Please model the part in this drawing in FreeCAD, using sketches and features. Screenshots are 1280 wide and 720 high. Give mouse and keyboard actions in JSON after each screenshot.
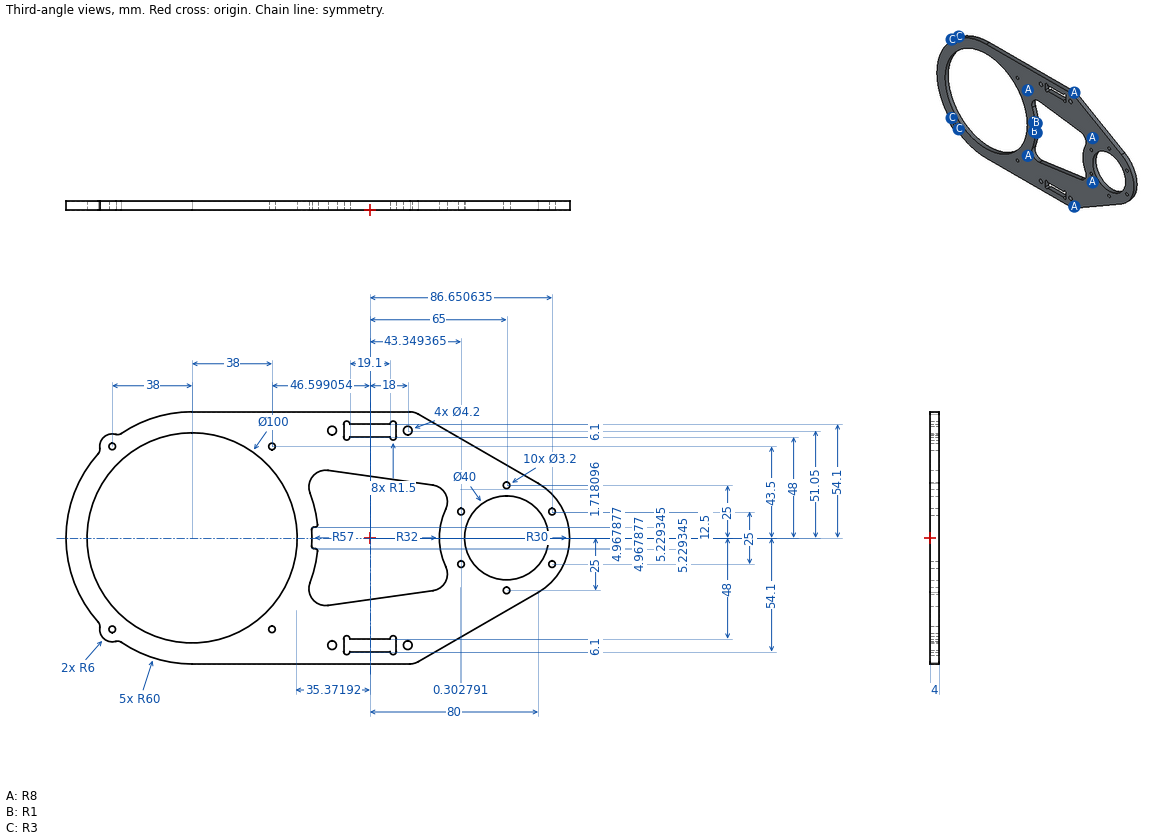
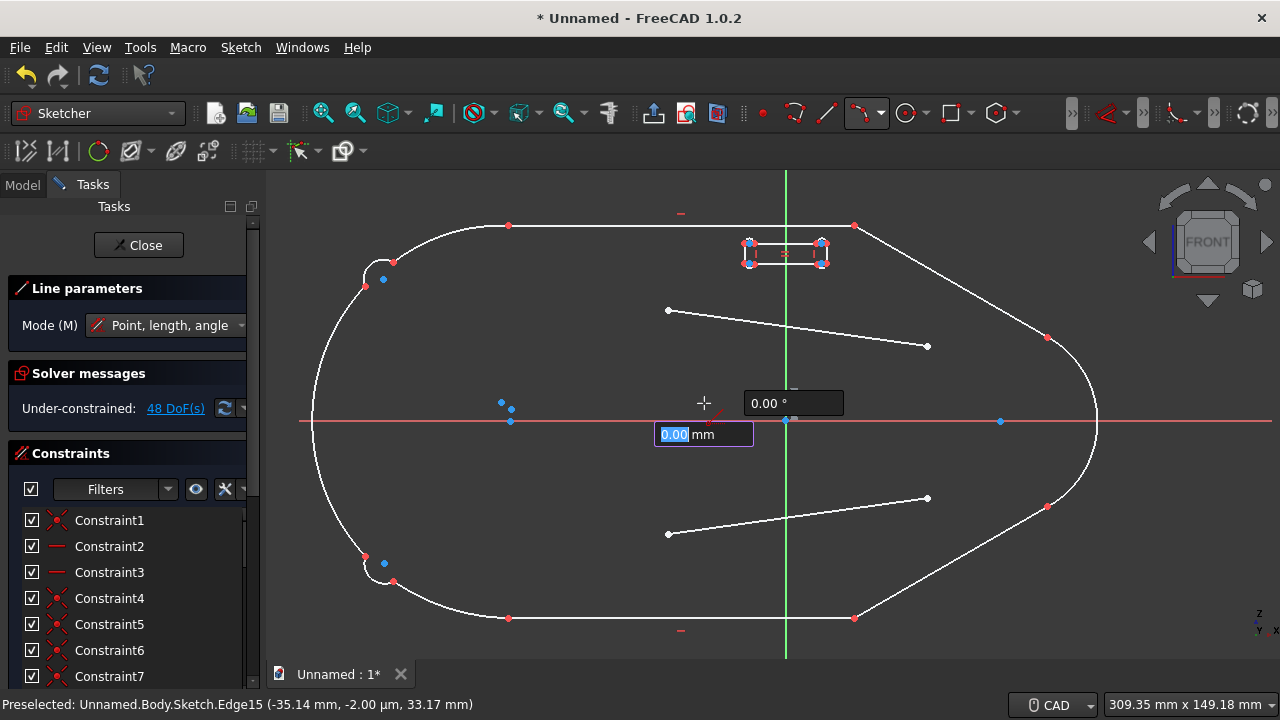
{"action": "scroll", "coordinate": [694, 404], "scroll_direction": "up", "scroll_amount": 3}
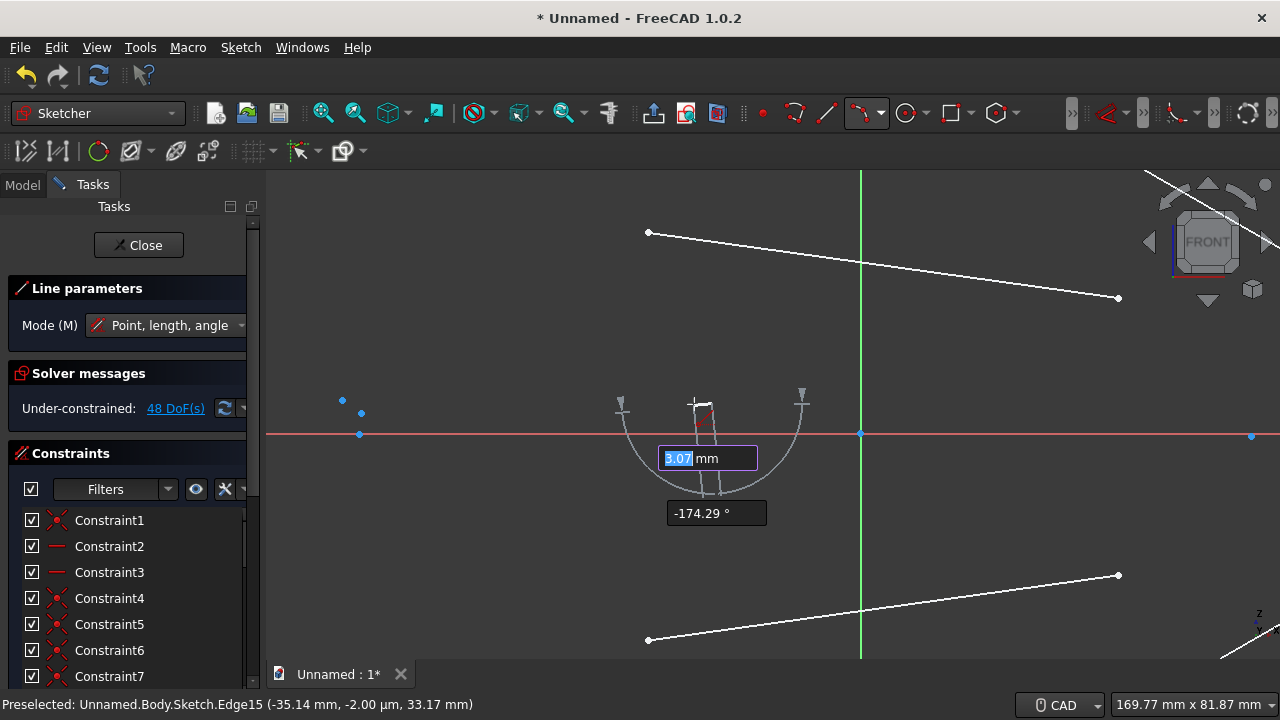
{"action": "left_click", "coordinate": [695, 404]}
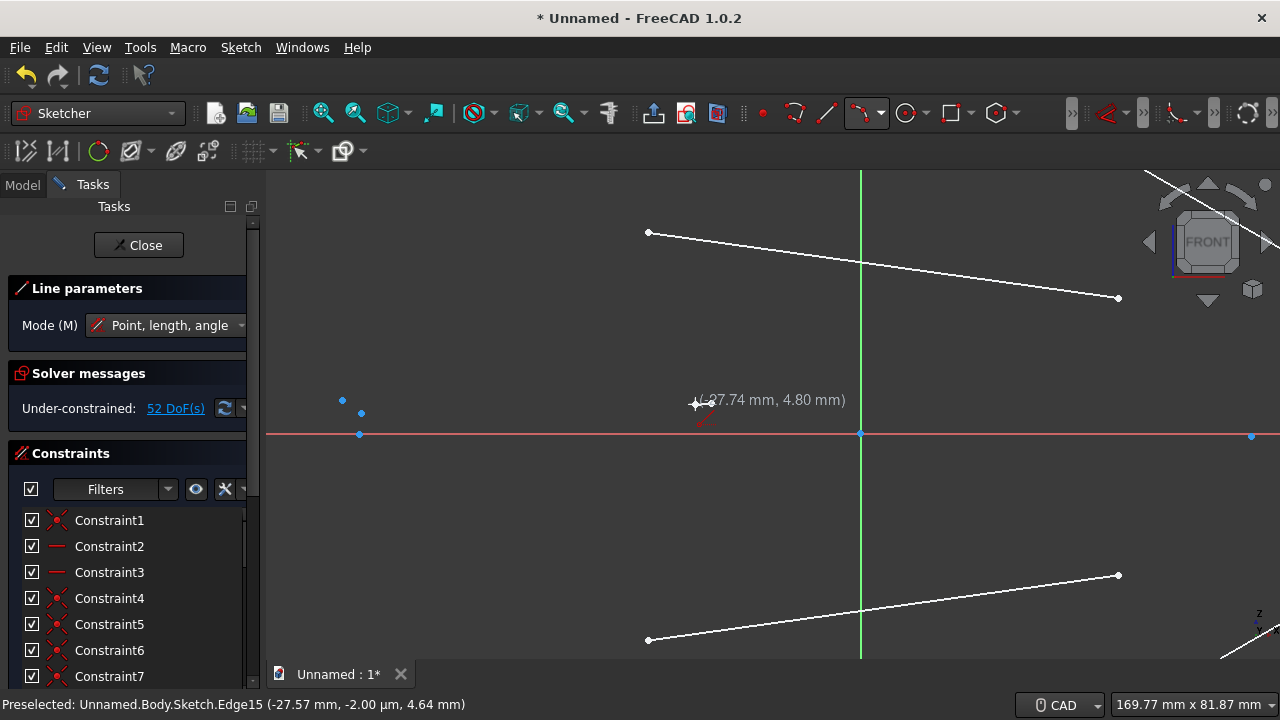
{"action": "left_click", "coordinate": [695, 463]}
{"action": "left_click", "coordinate": [712, 465]}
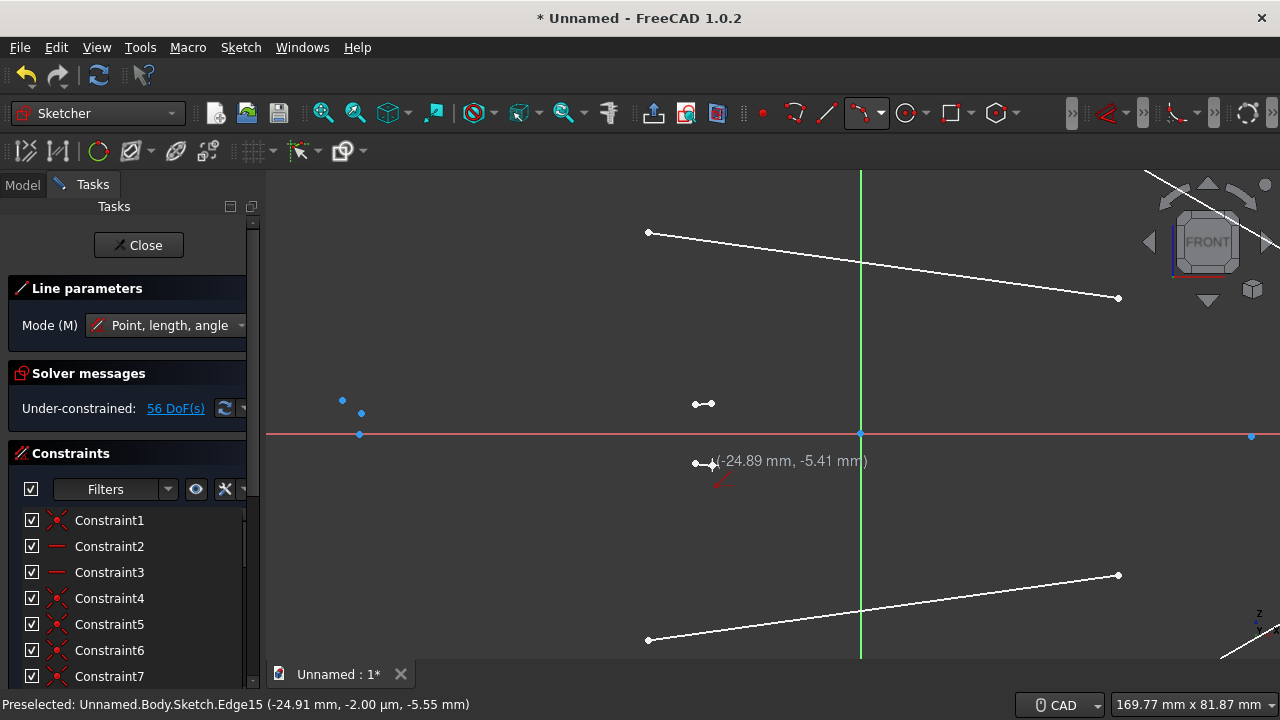
{"action": "left_click", "coordinate": [860, 114]}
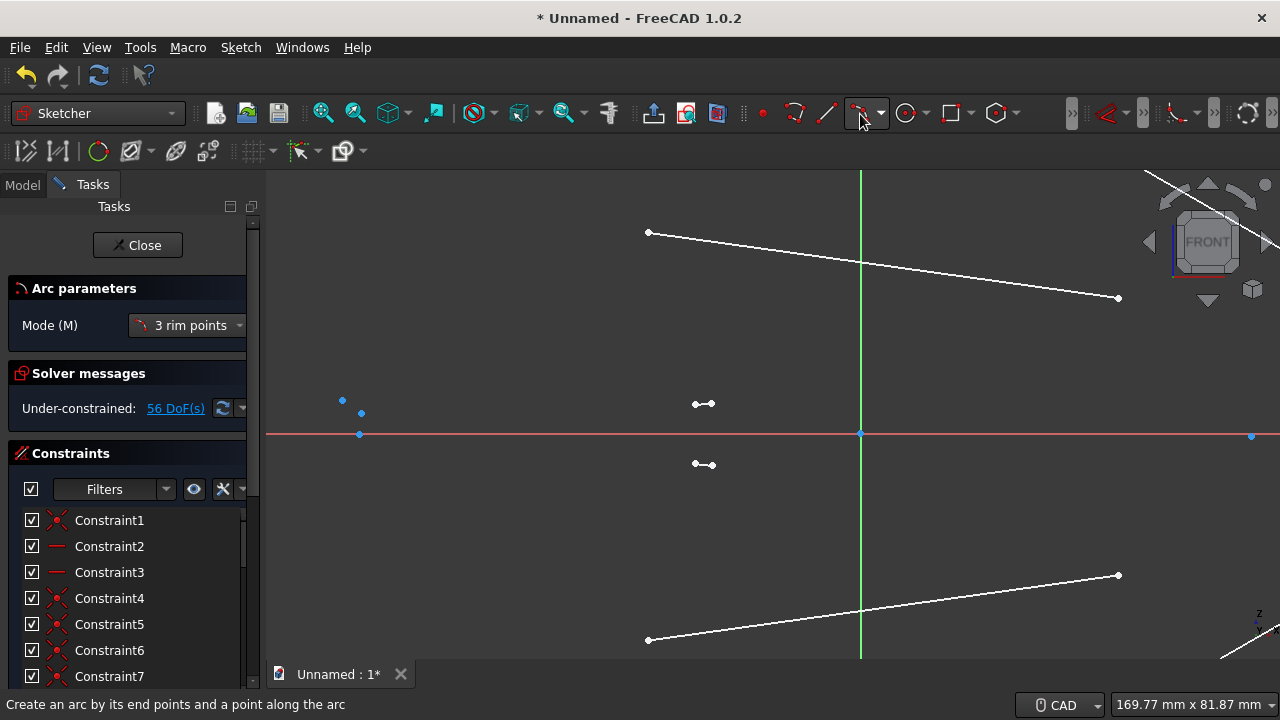
{"action": "scroll", "coordinate": [700, 403], "scroll_direction": "down", "scroll_amount": 5}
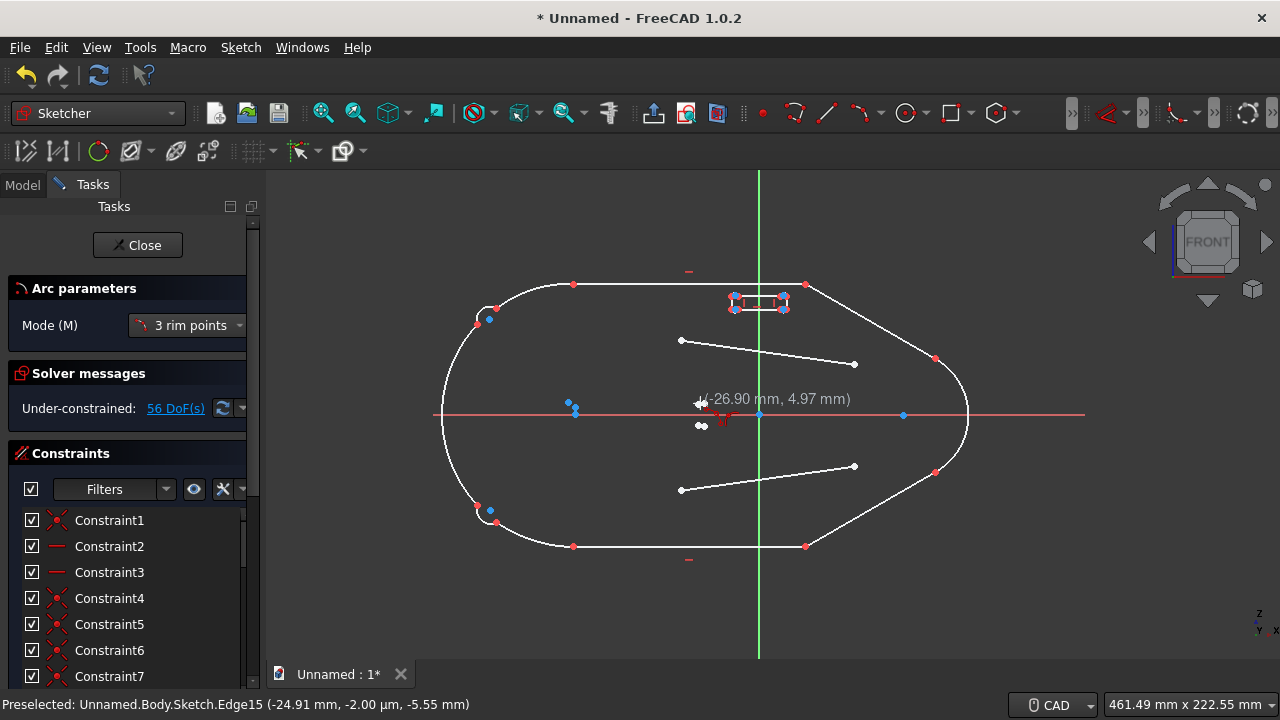
{"action": "left_click", "coordinate": [854, 467]}
{"action": "left_click", "coordinate": [854, 365]}
{"action": "left_click", "coordinate": [836, 392]}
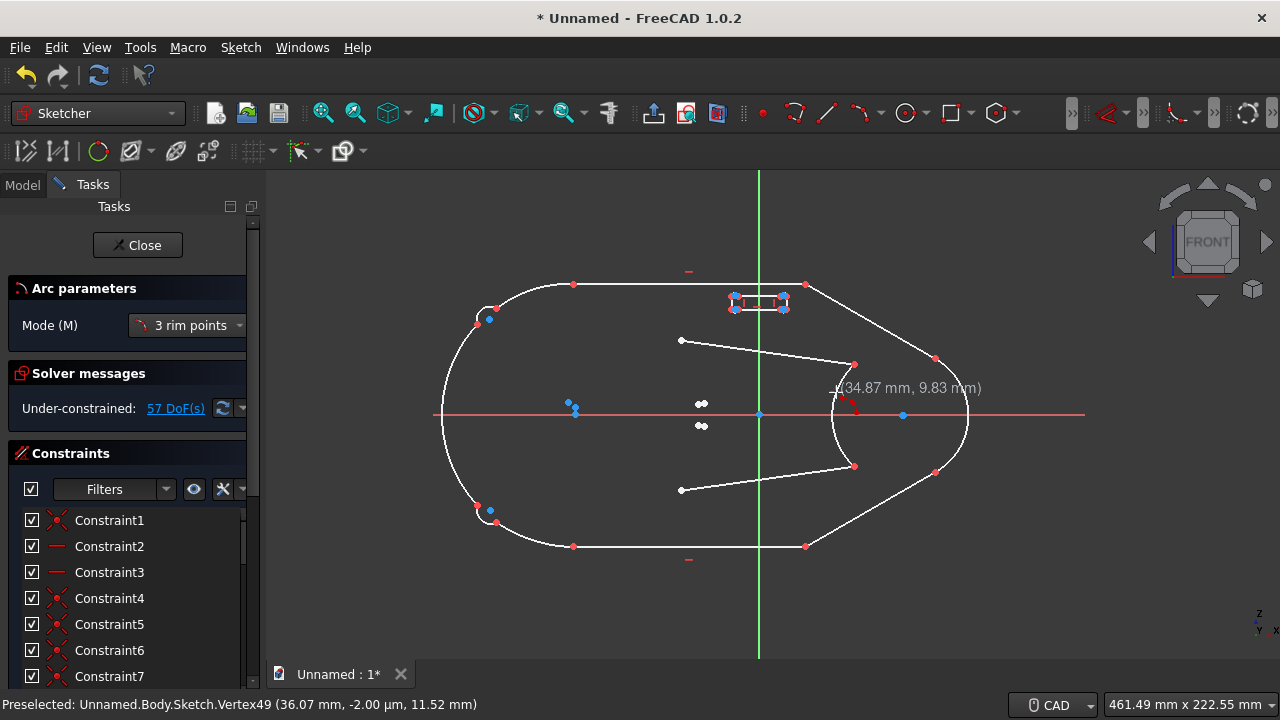
{"action": "left_click", "coordinate": [681, 341]}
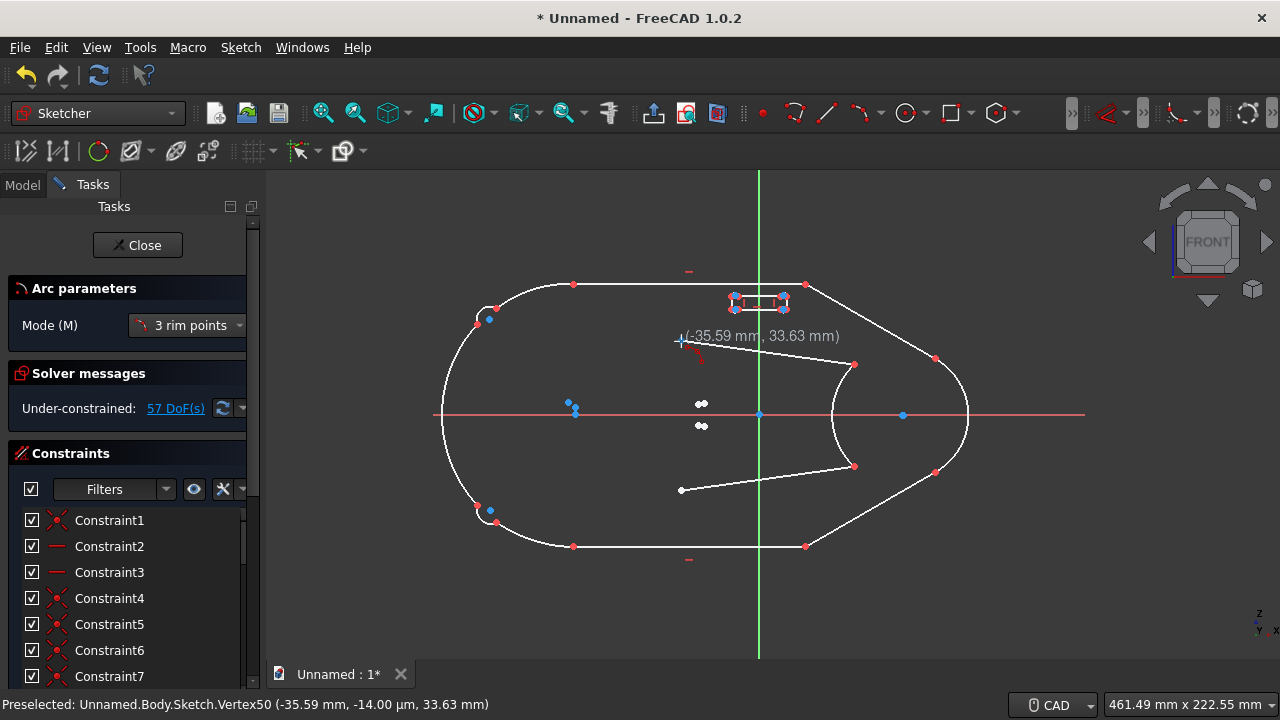
{"action": "scroll", "coordinate": [705, 403], "scroll_direction": "up", "scroll_amount": 8}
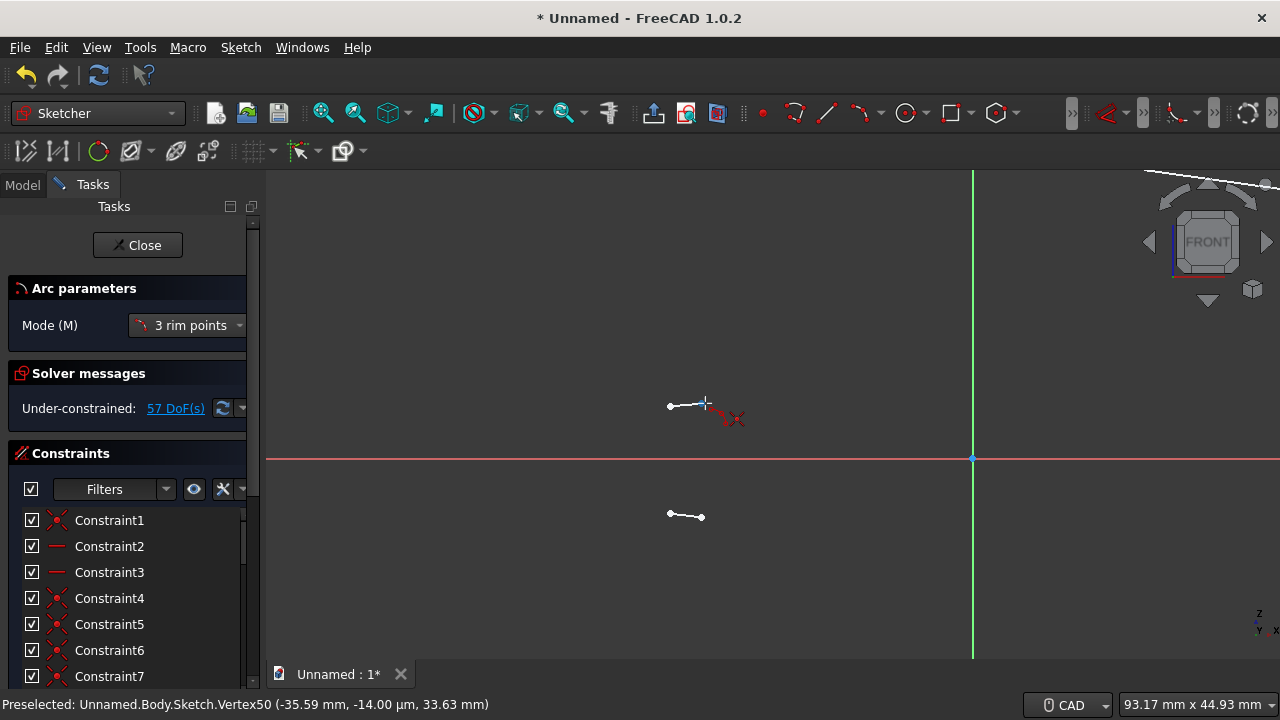
{"action": "left_click", "coordinate": [701, 404]}
{"action": "left_click", "coordinate": [666, 236]}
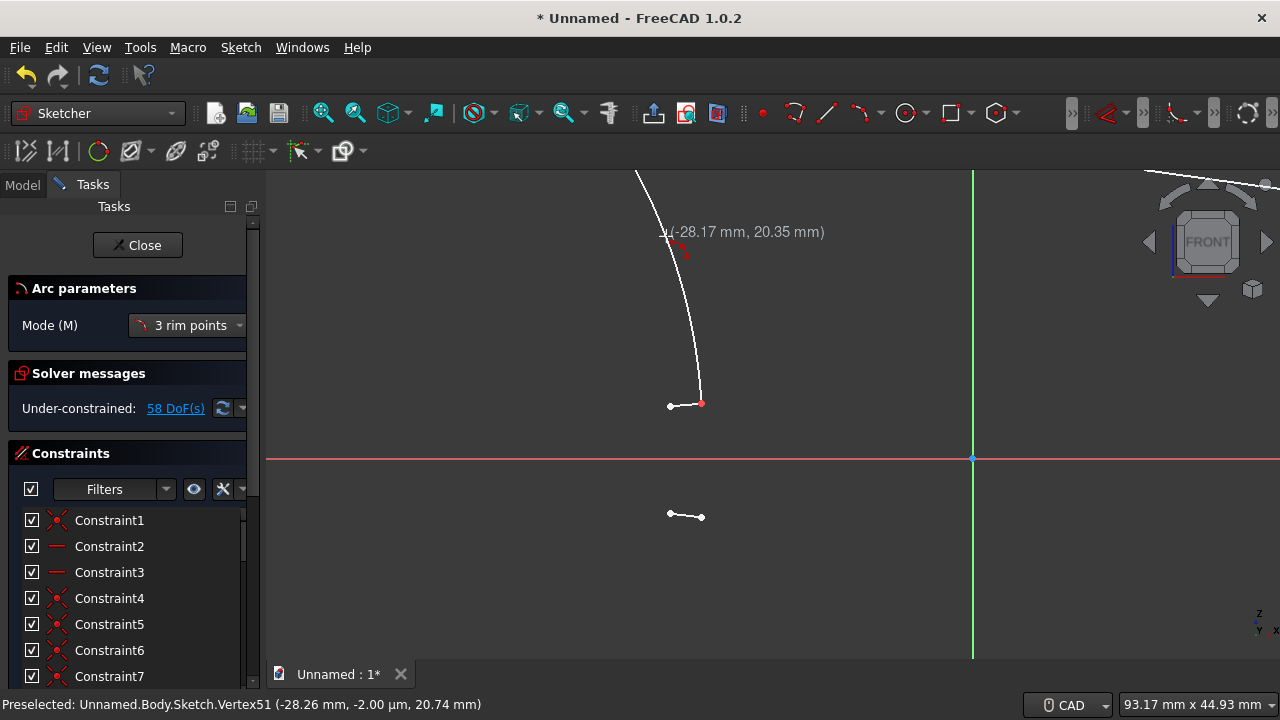
{"action": "left_click", "coordinate": [671, 406]}
{"action": "left_click", "coordinate": [671, 514]}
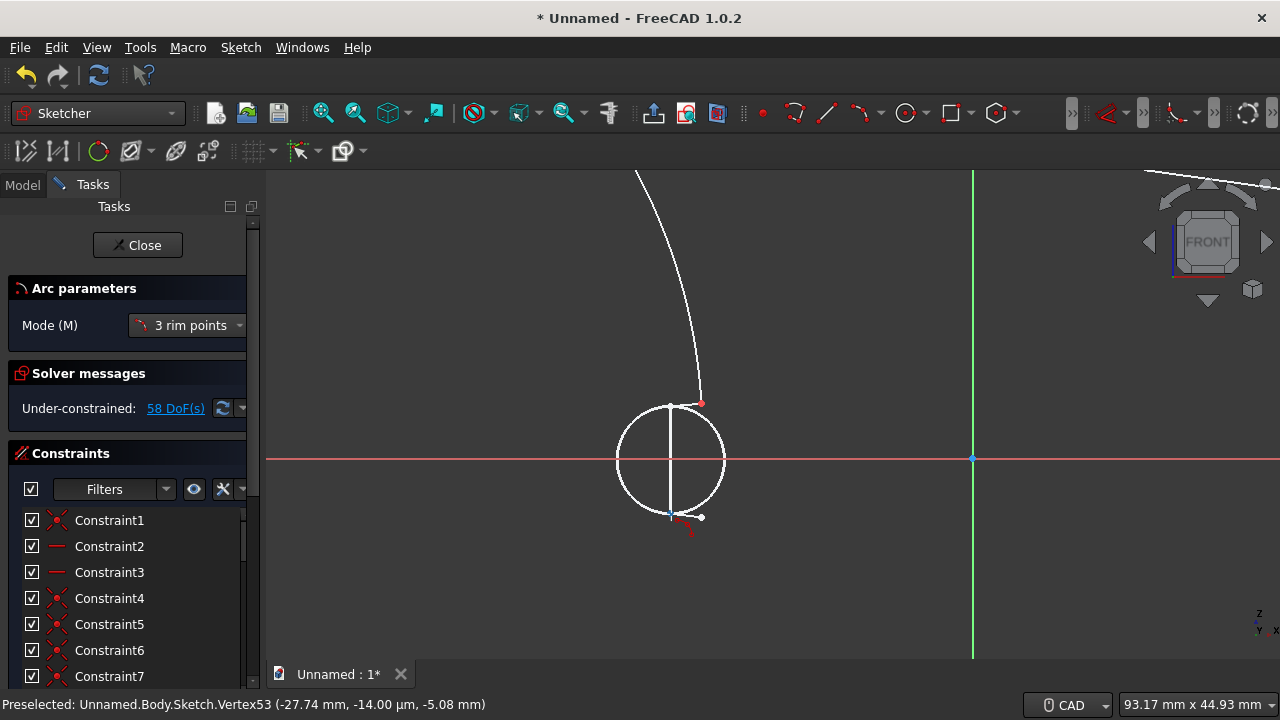
{"action": "scroll", "coordinate": [672, 469], "scroll_direction": "up", "scroll_amount": 10}